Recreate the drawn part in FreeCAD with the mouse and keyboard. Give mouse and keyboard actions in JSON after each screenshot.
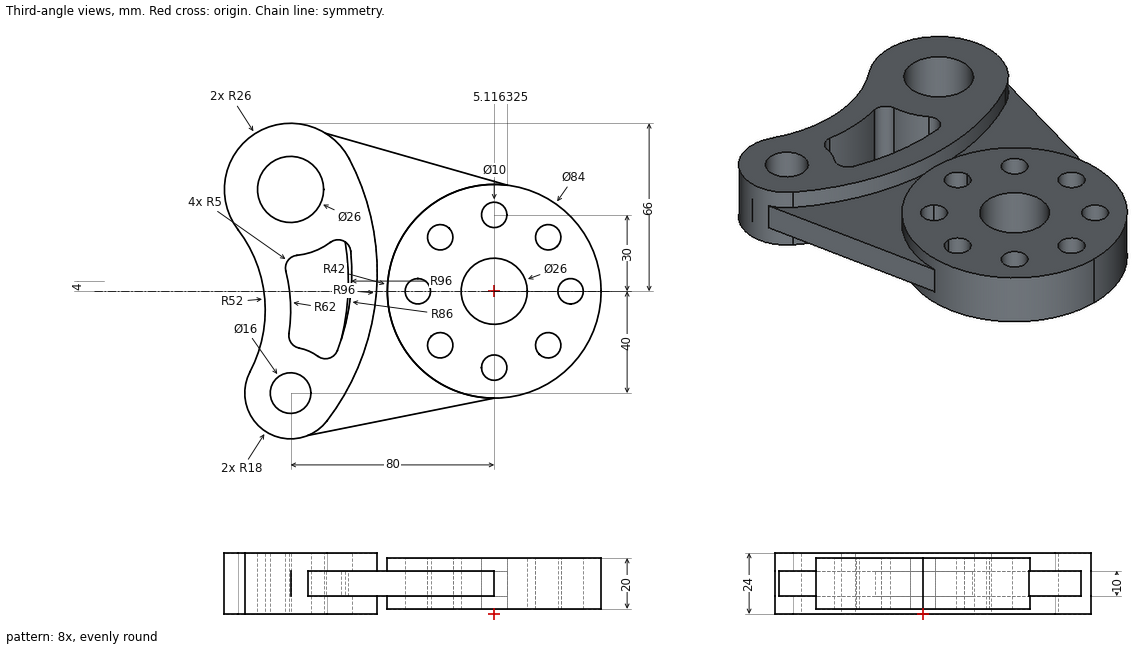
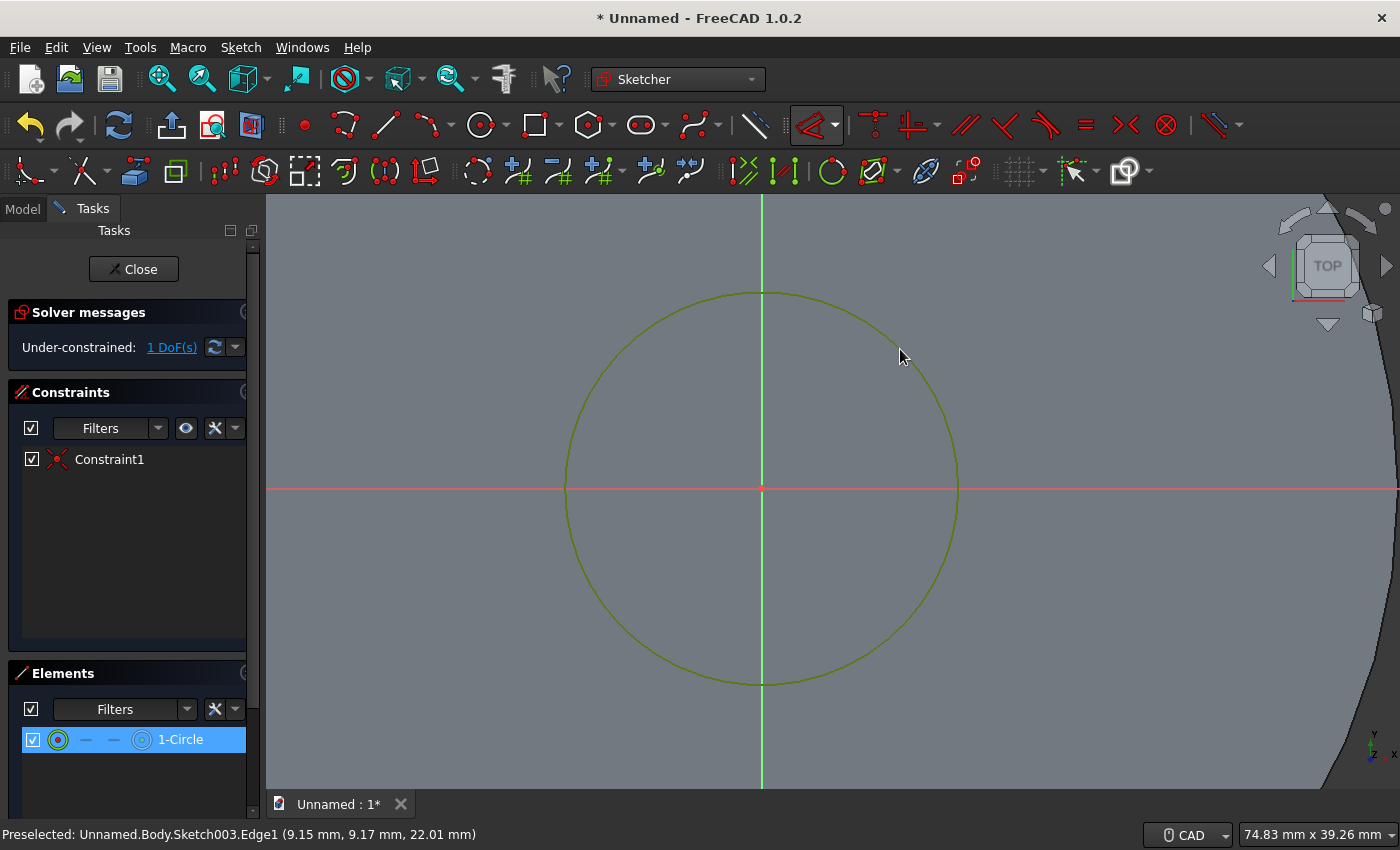
{"action": "left_click", "coordinate": [838, 126]}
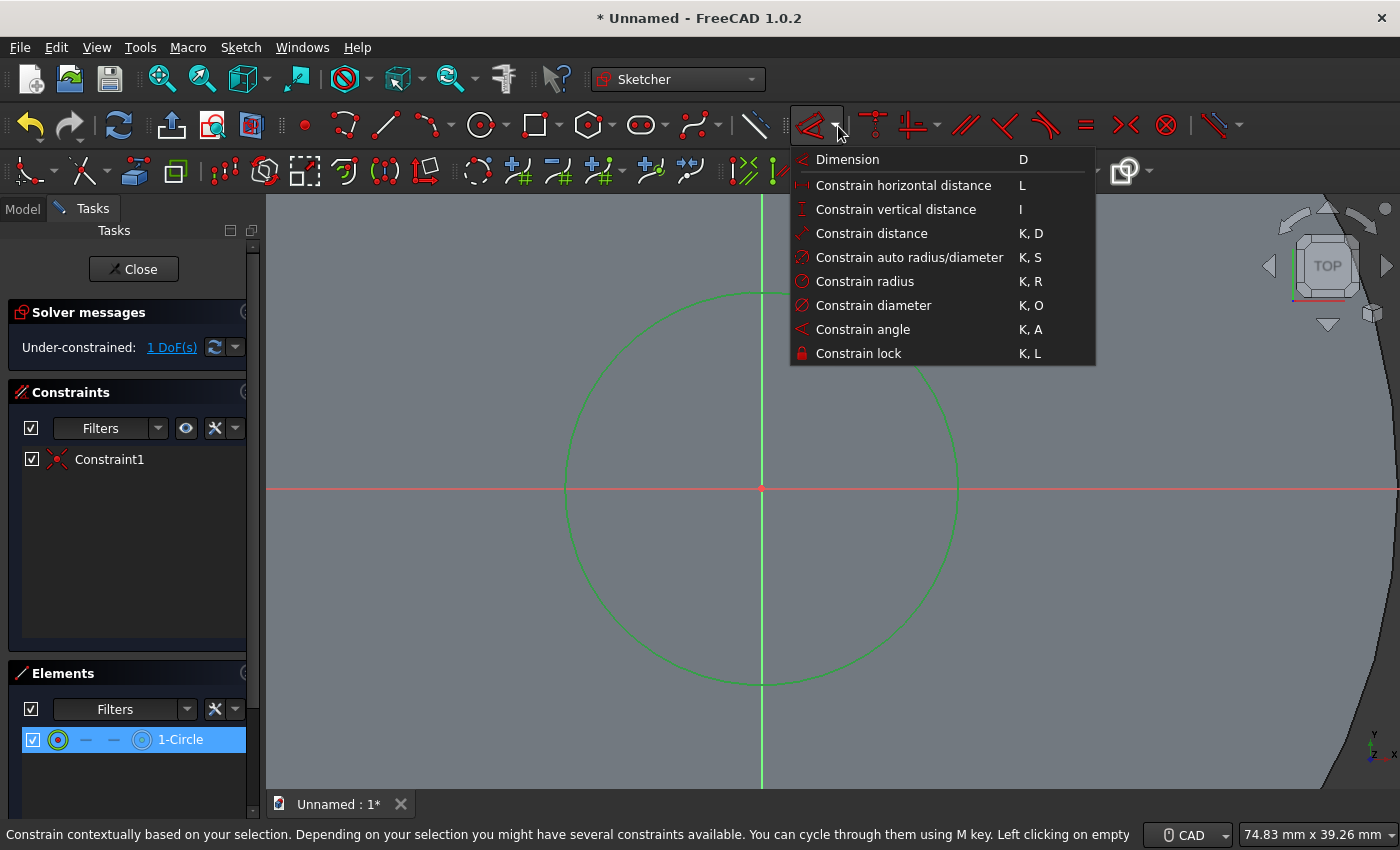
{"action": "left_click", "coordinate": [943, 305]}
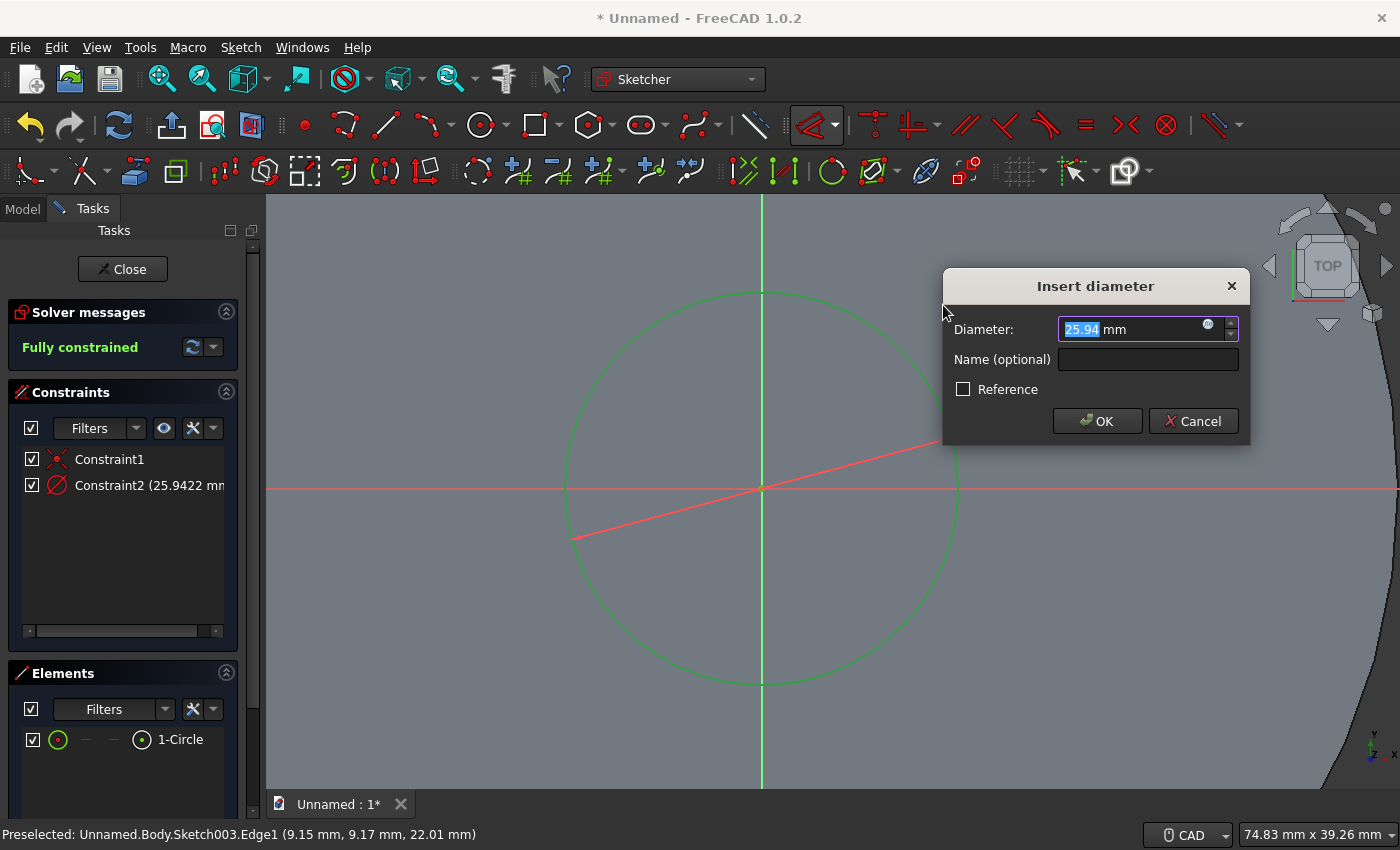
{"action": "type", "text": "26"}
{"action": "key", "text": "Return"}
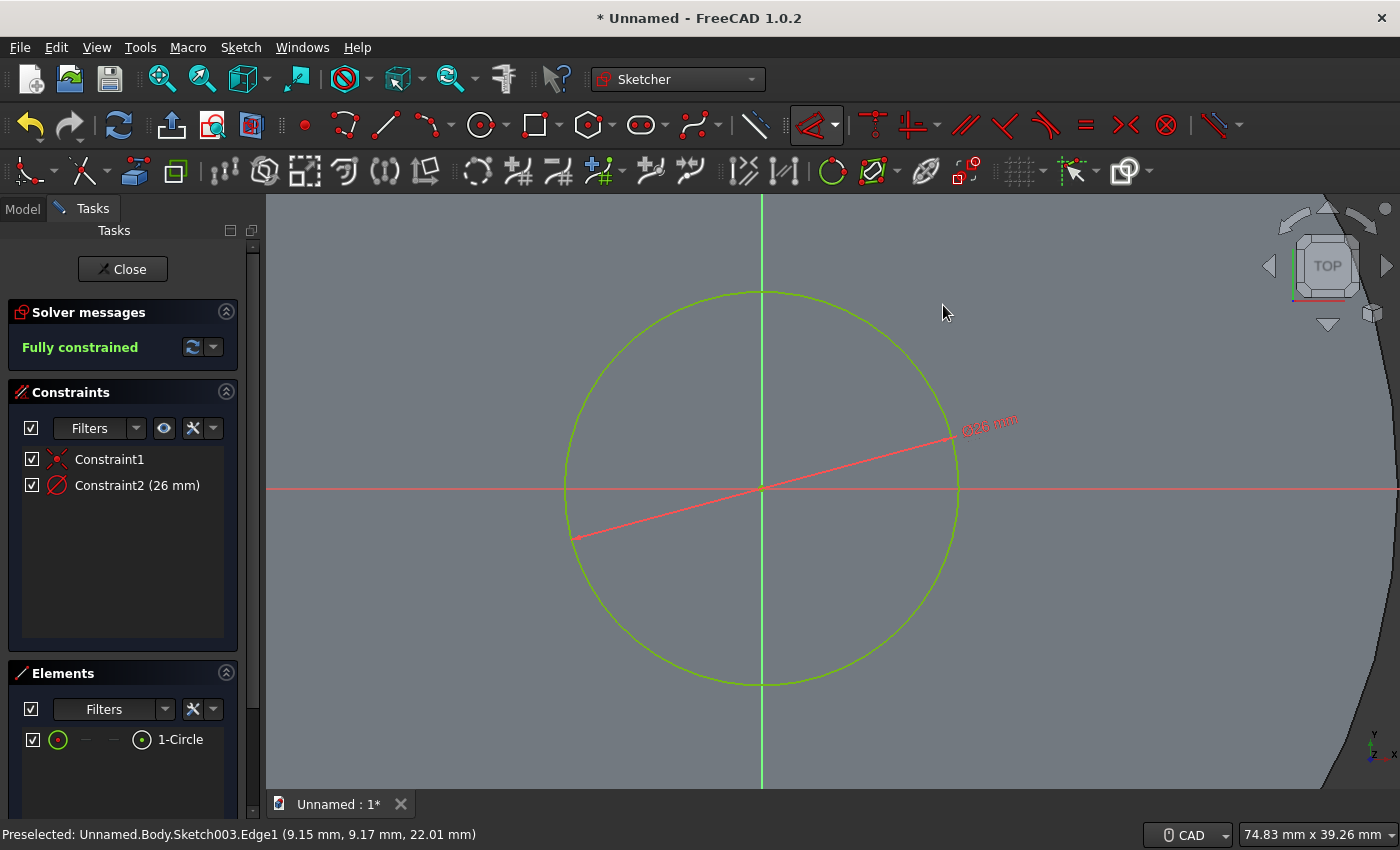
{"action": "left_click", "coordinate": [123, 269]}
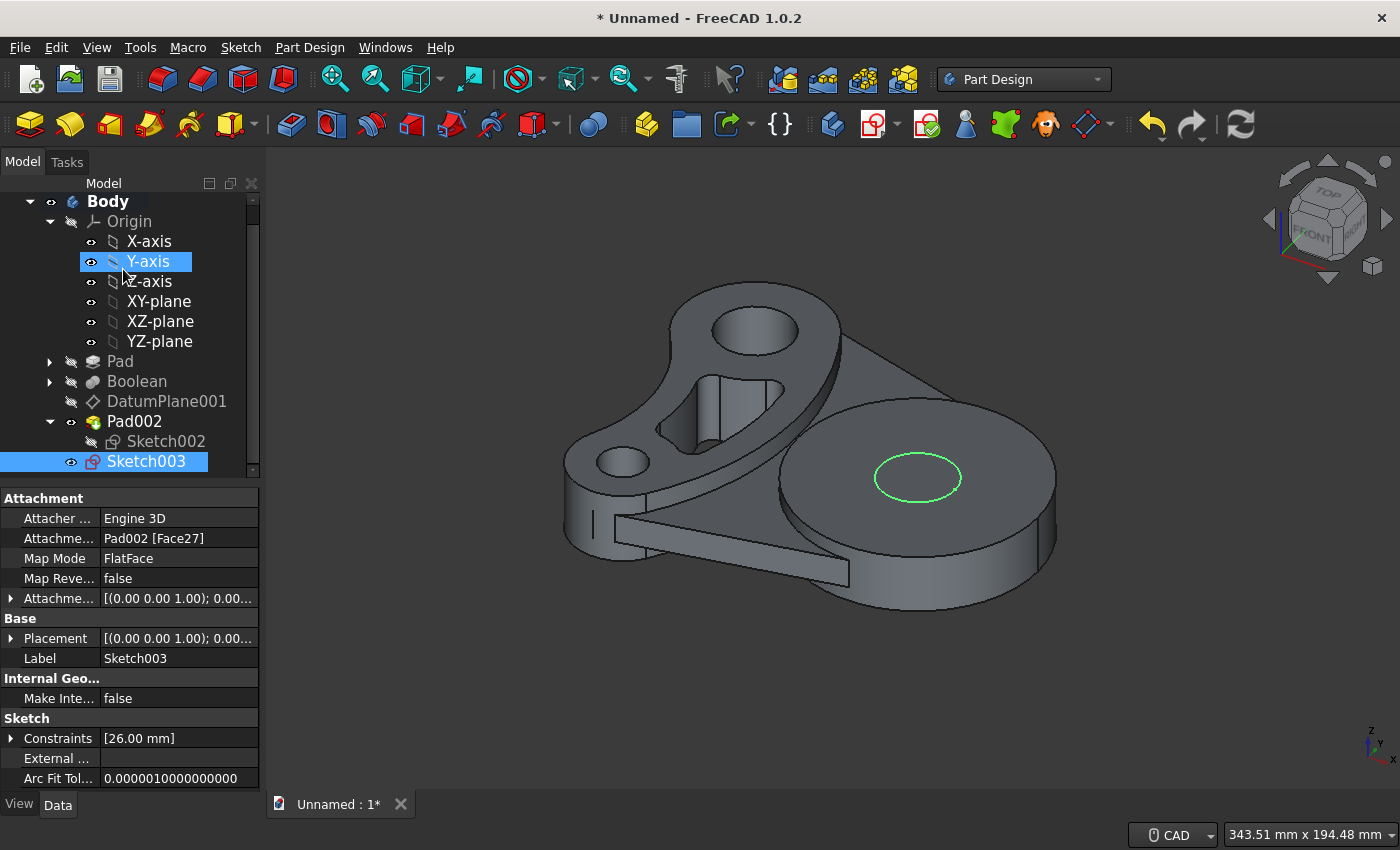
{"action": "left_click", "coordinate": [292, 124]}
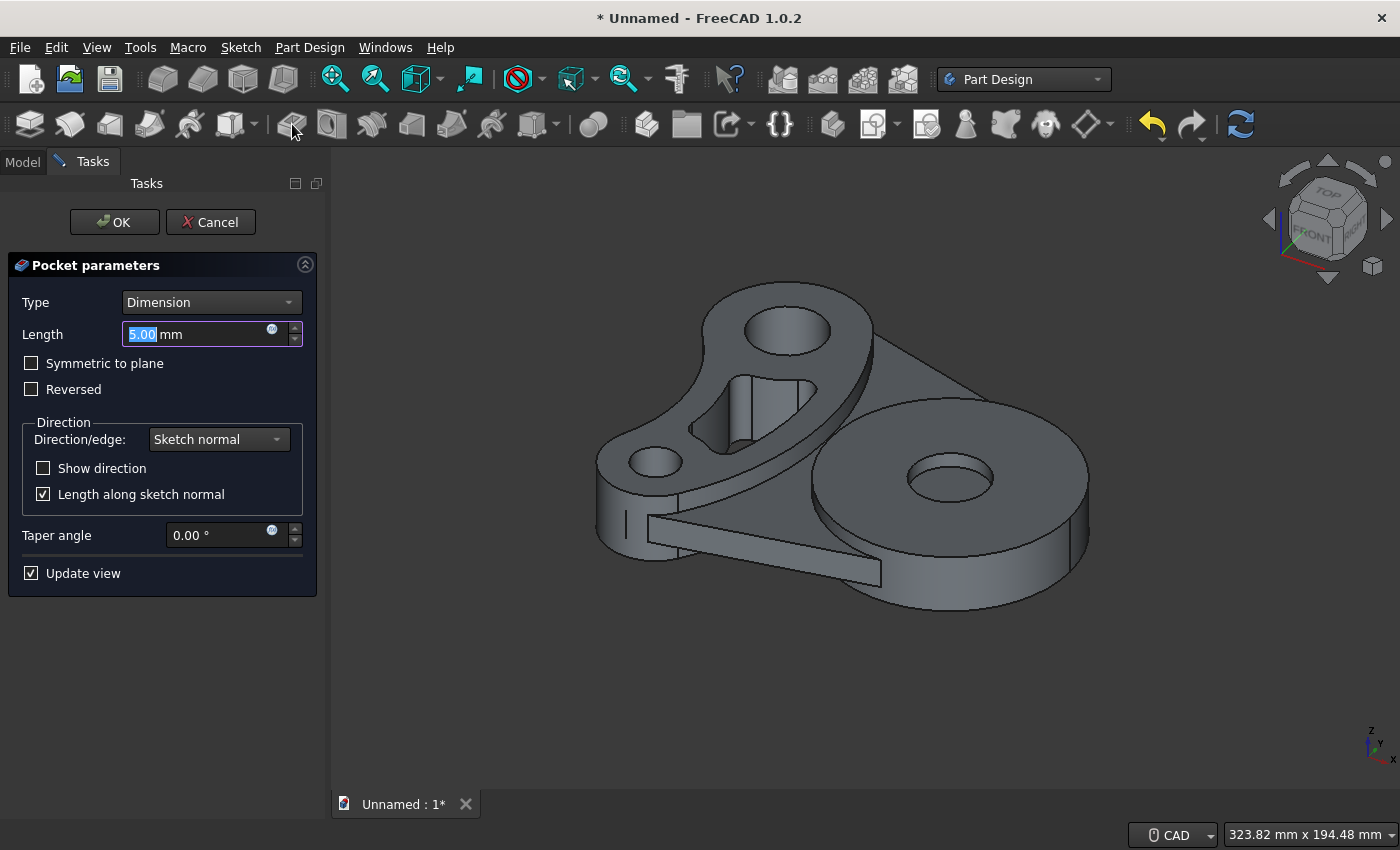
{"action": "left_click", "coordinate": [212, 302]}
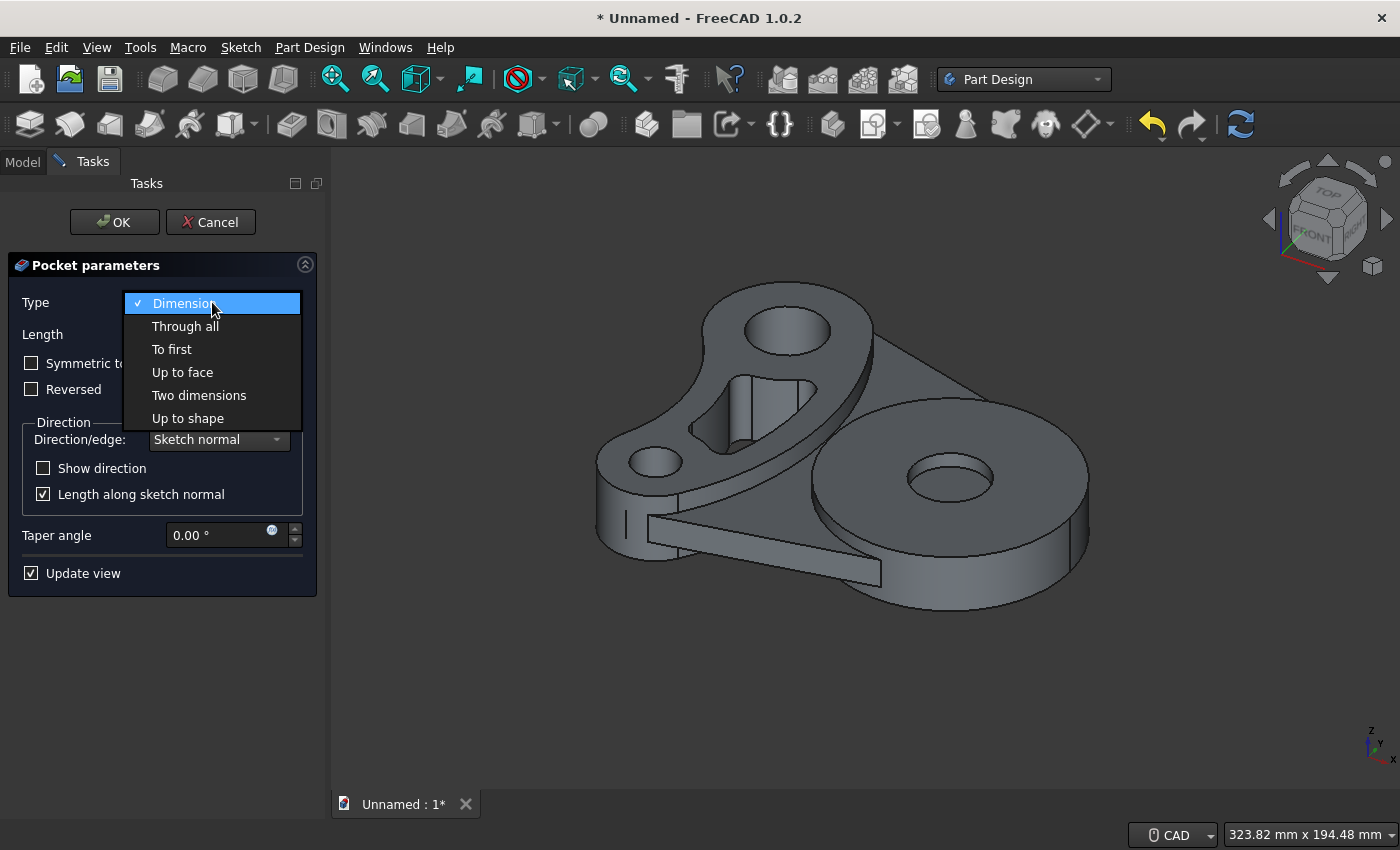
{"action": "left_click", "coordinate": [212, 326]}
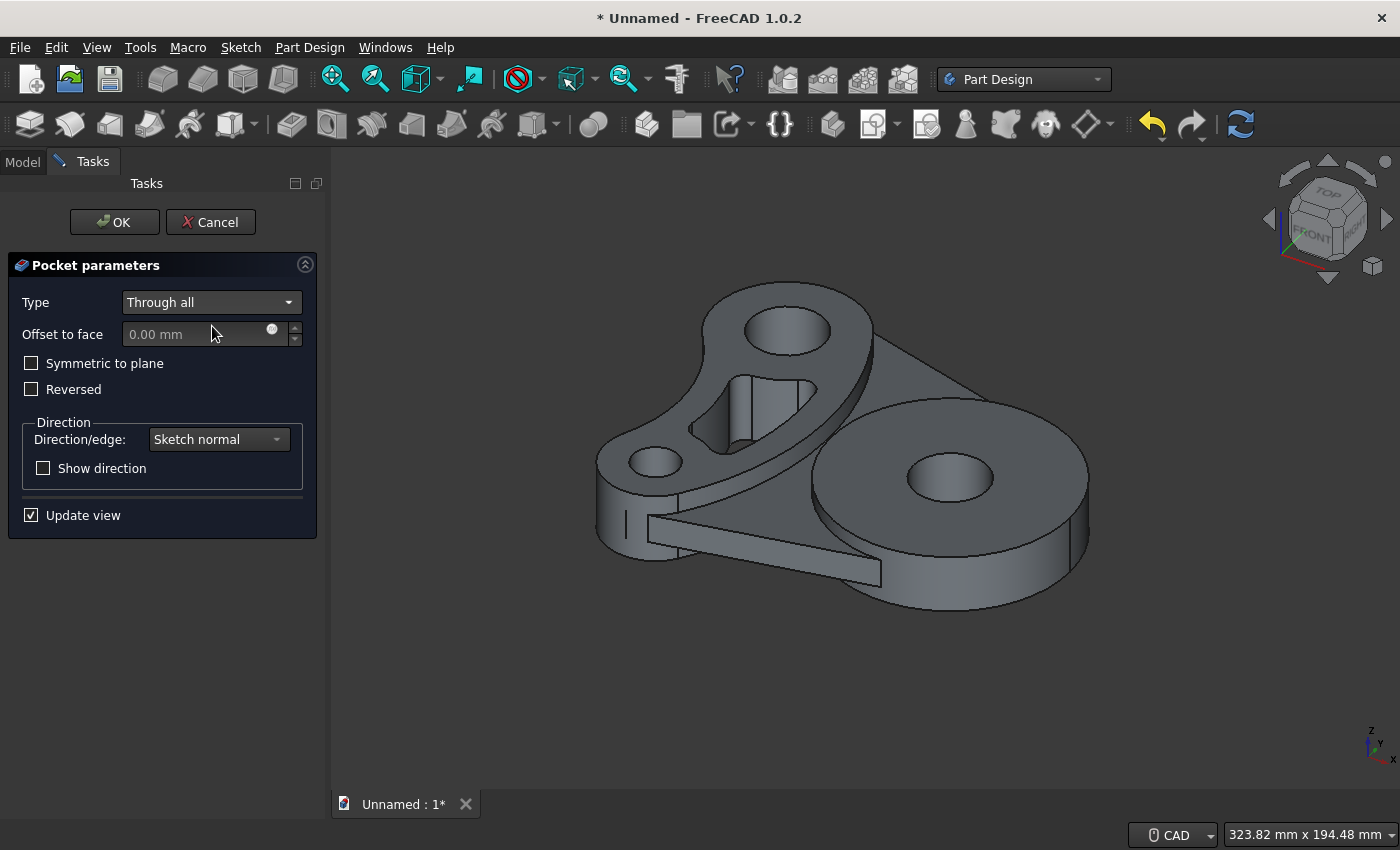
{"action": "left_click", "coordinate": [115, 222]}